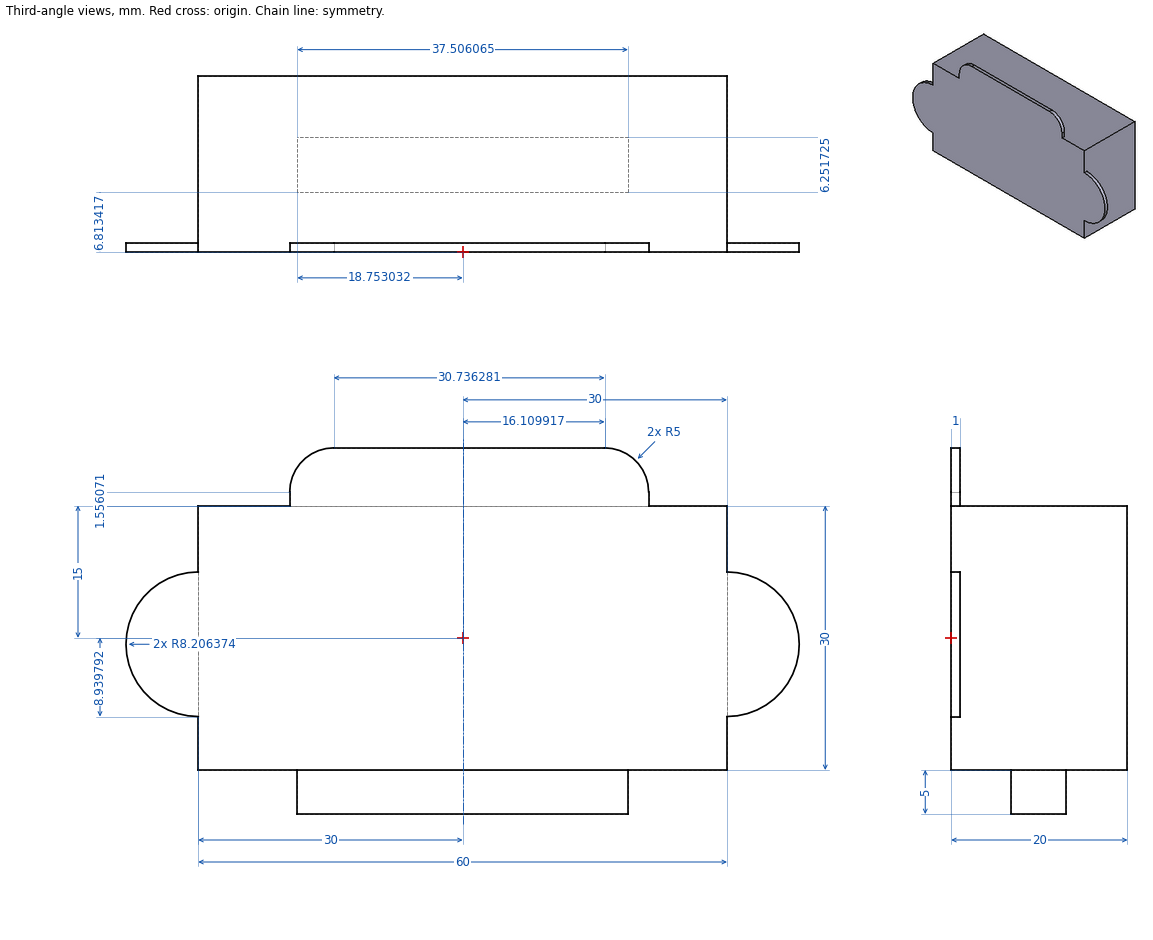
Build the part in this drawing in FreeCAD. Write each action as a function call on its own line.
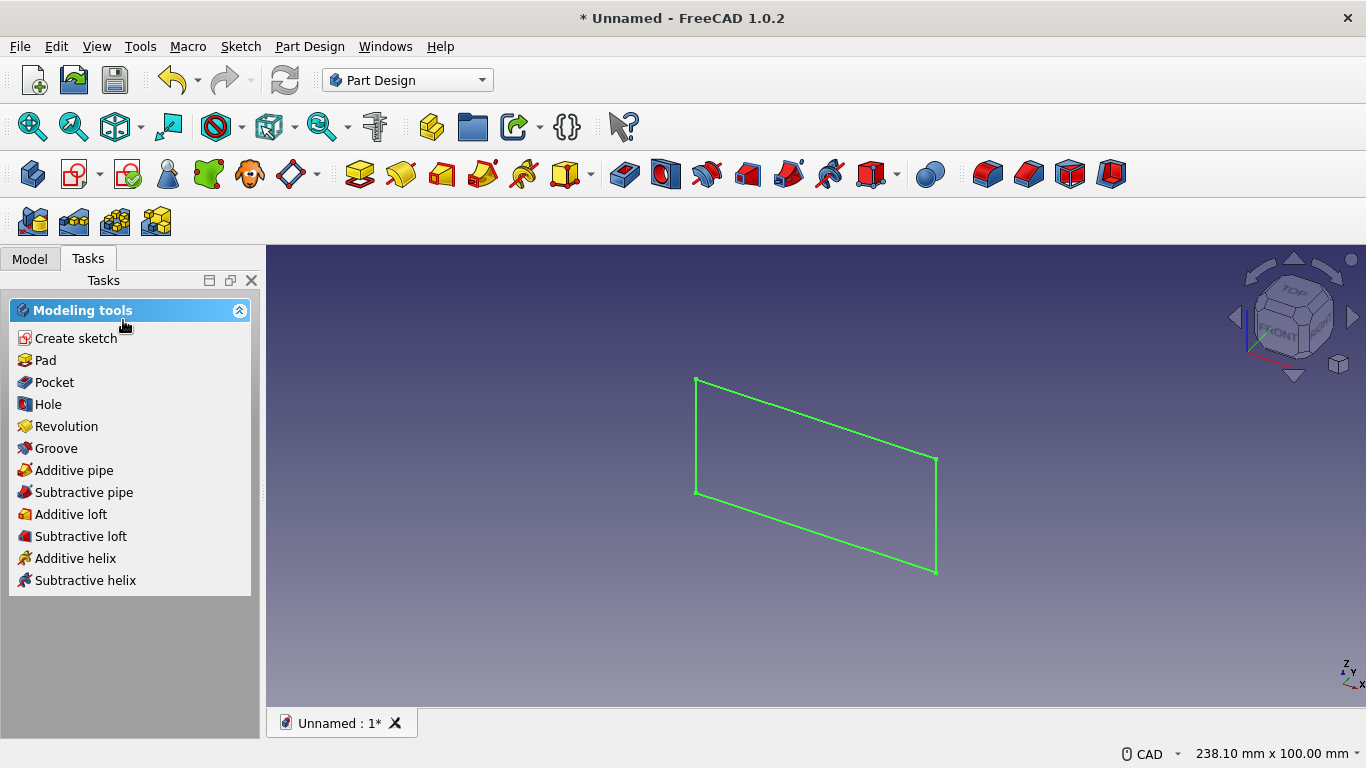
click(360, 174)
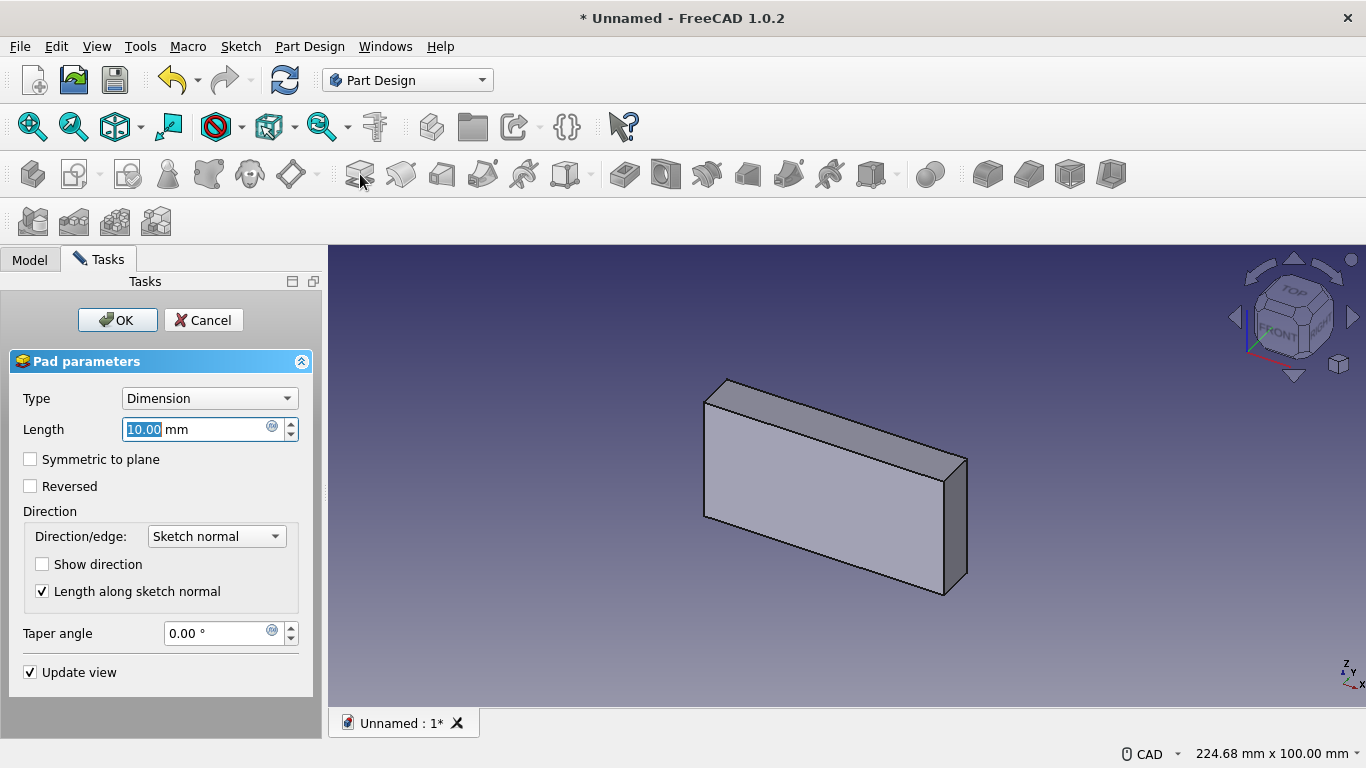
text(20)
key(Tab)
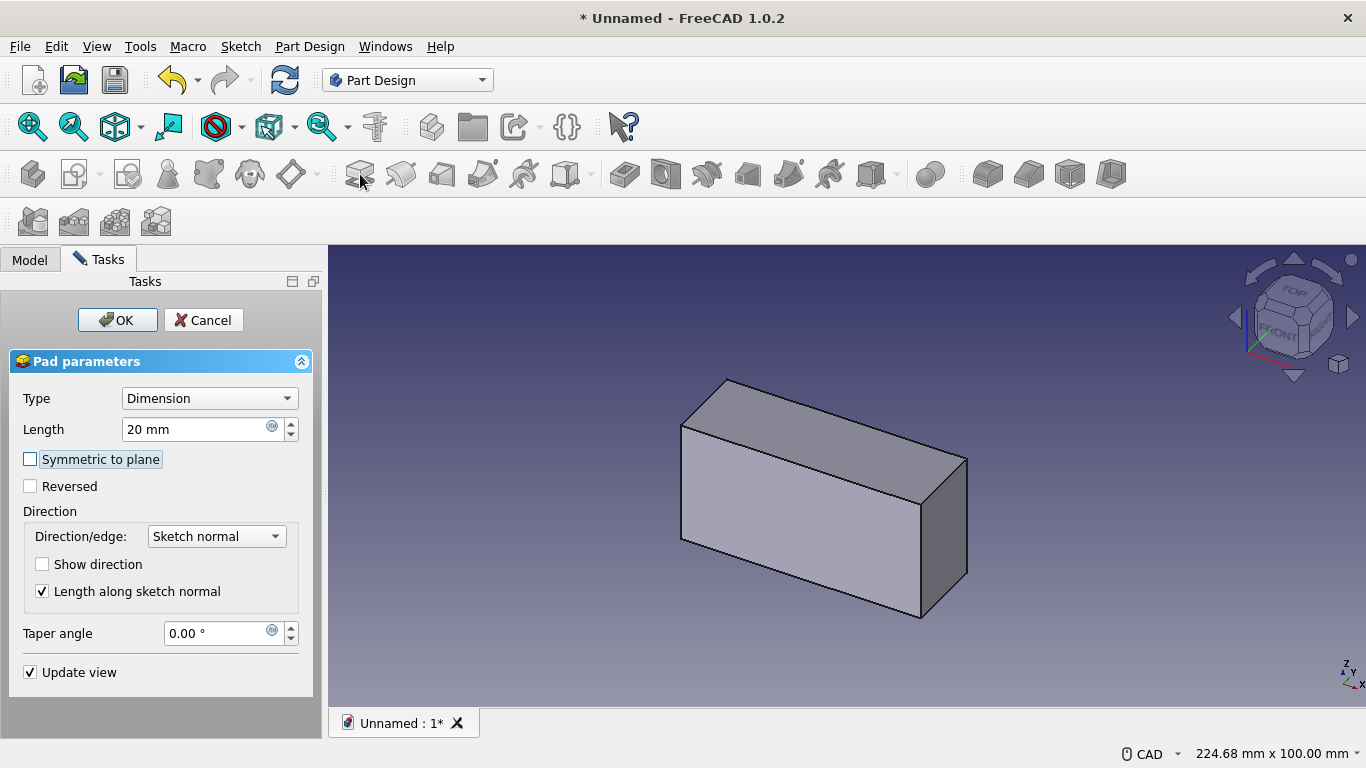
click(31, 486)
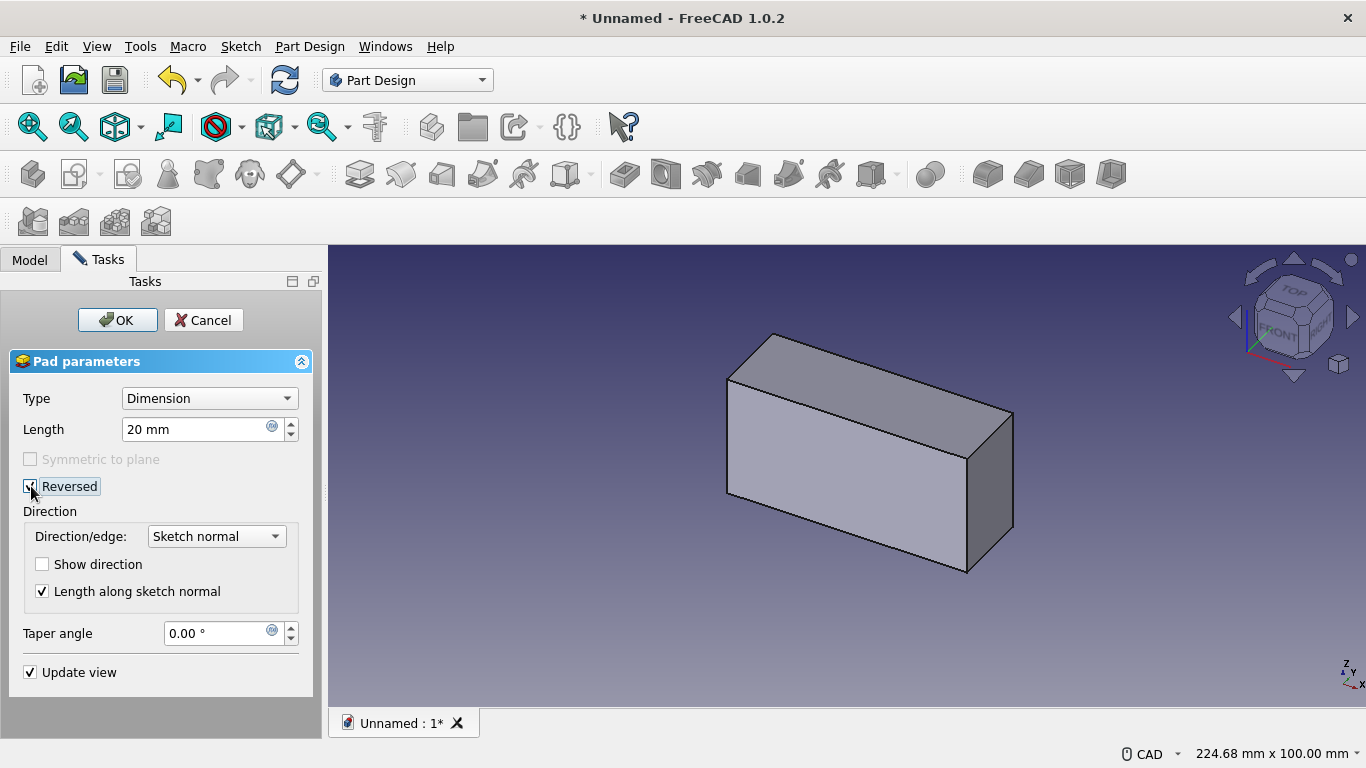
click(118, 320)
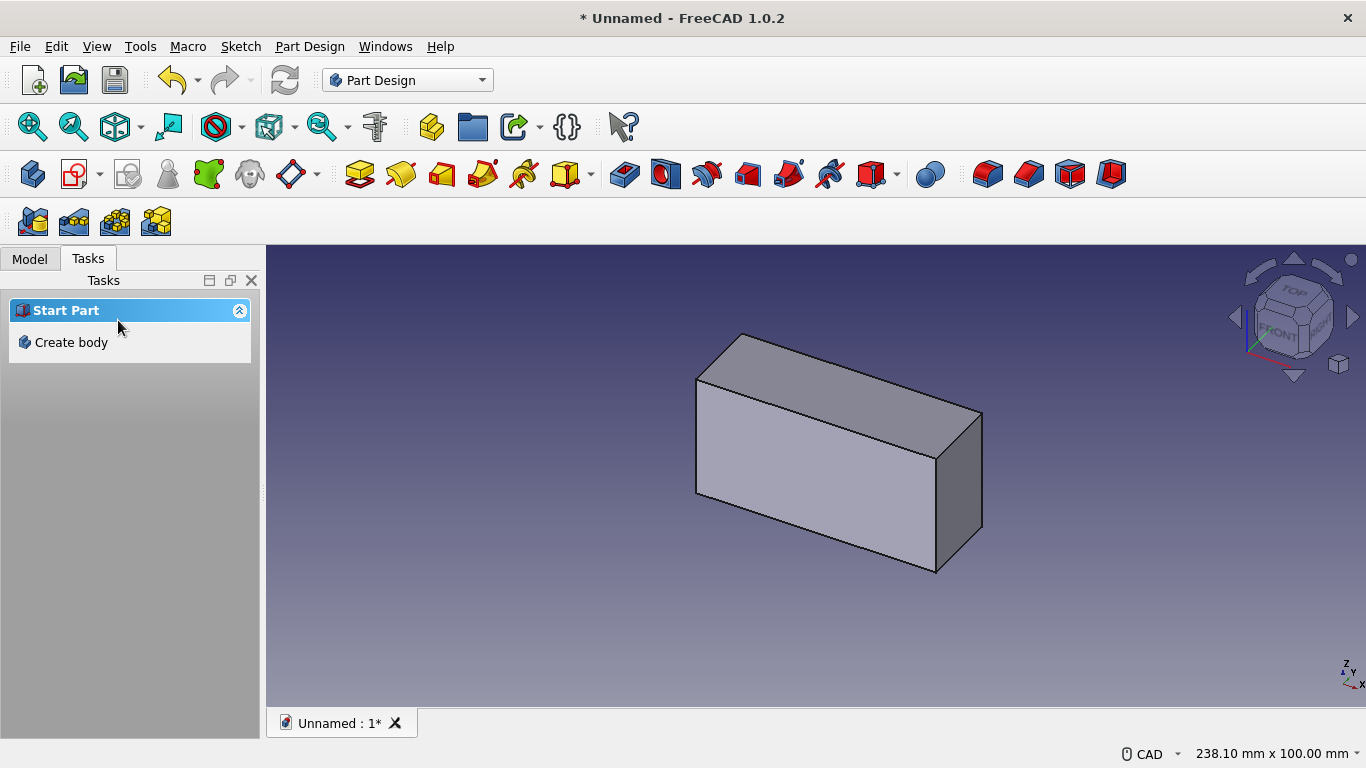
key(5)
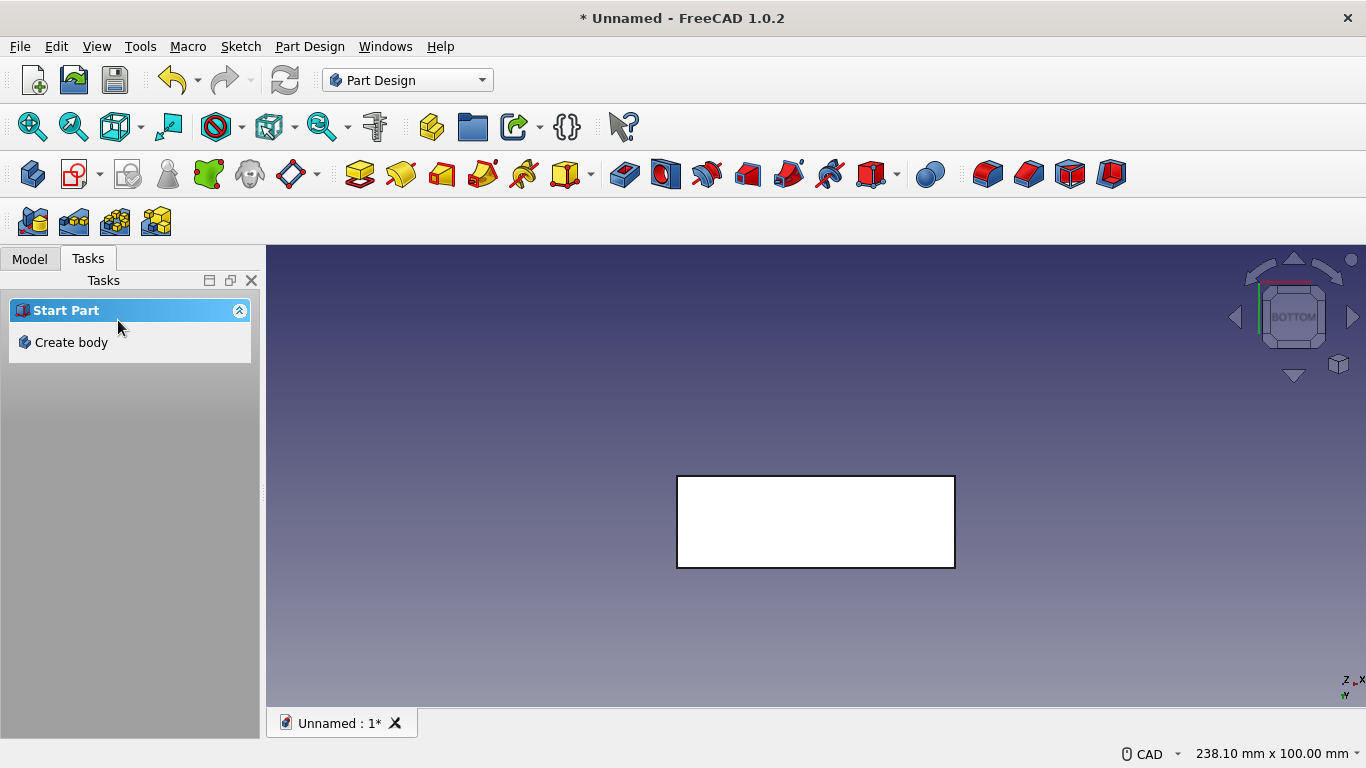
key(v)
key(f)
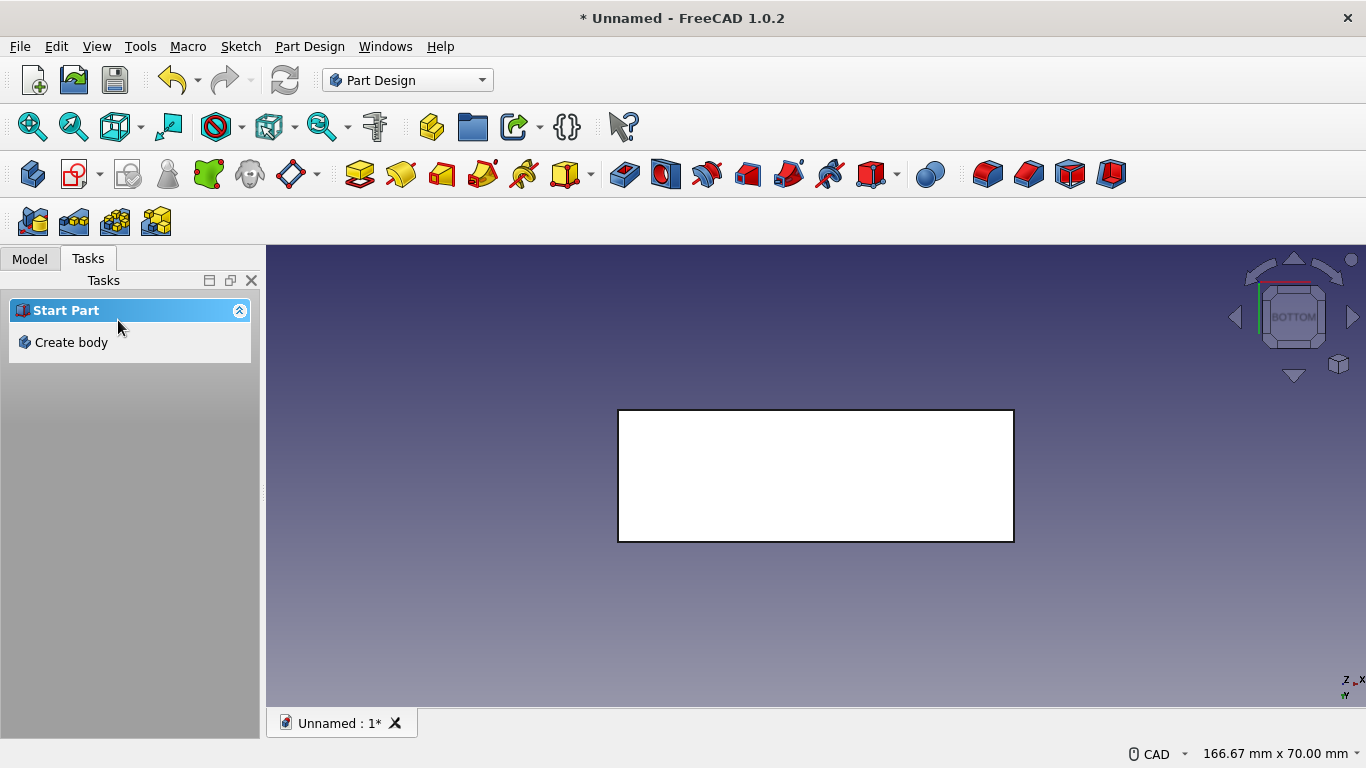
click(929, 475)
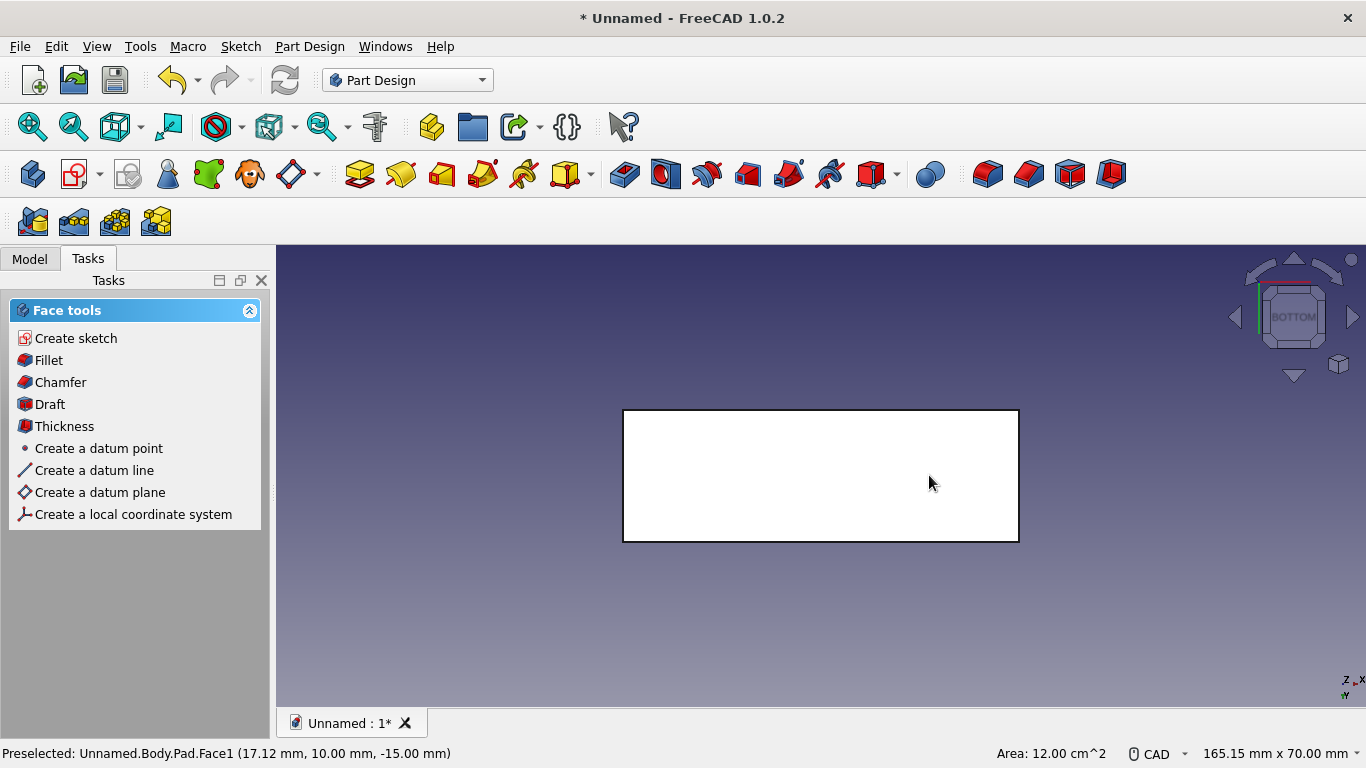
click(74, 174)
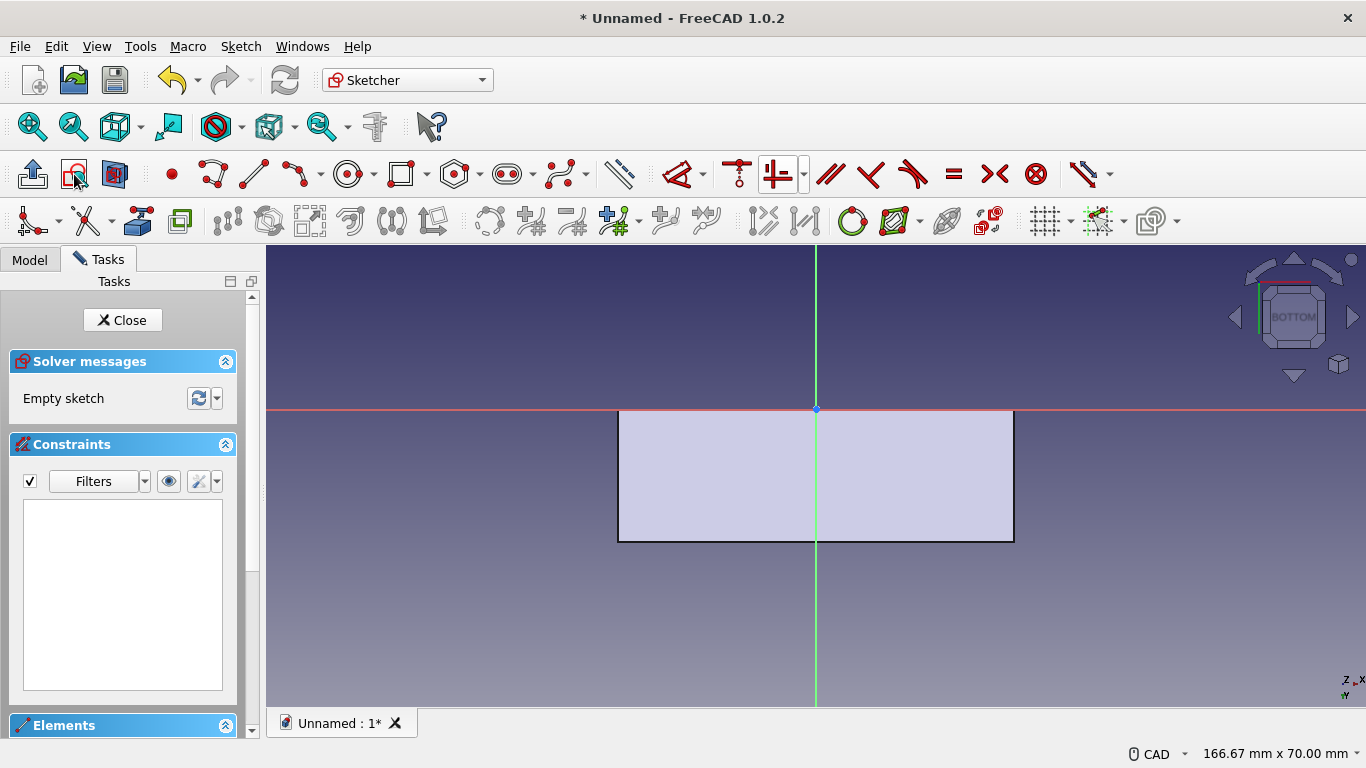
scroll(856, 440, up, 5)